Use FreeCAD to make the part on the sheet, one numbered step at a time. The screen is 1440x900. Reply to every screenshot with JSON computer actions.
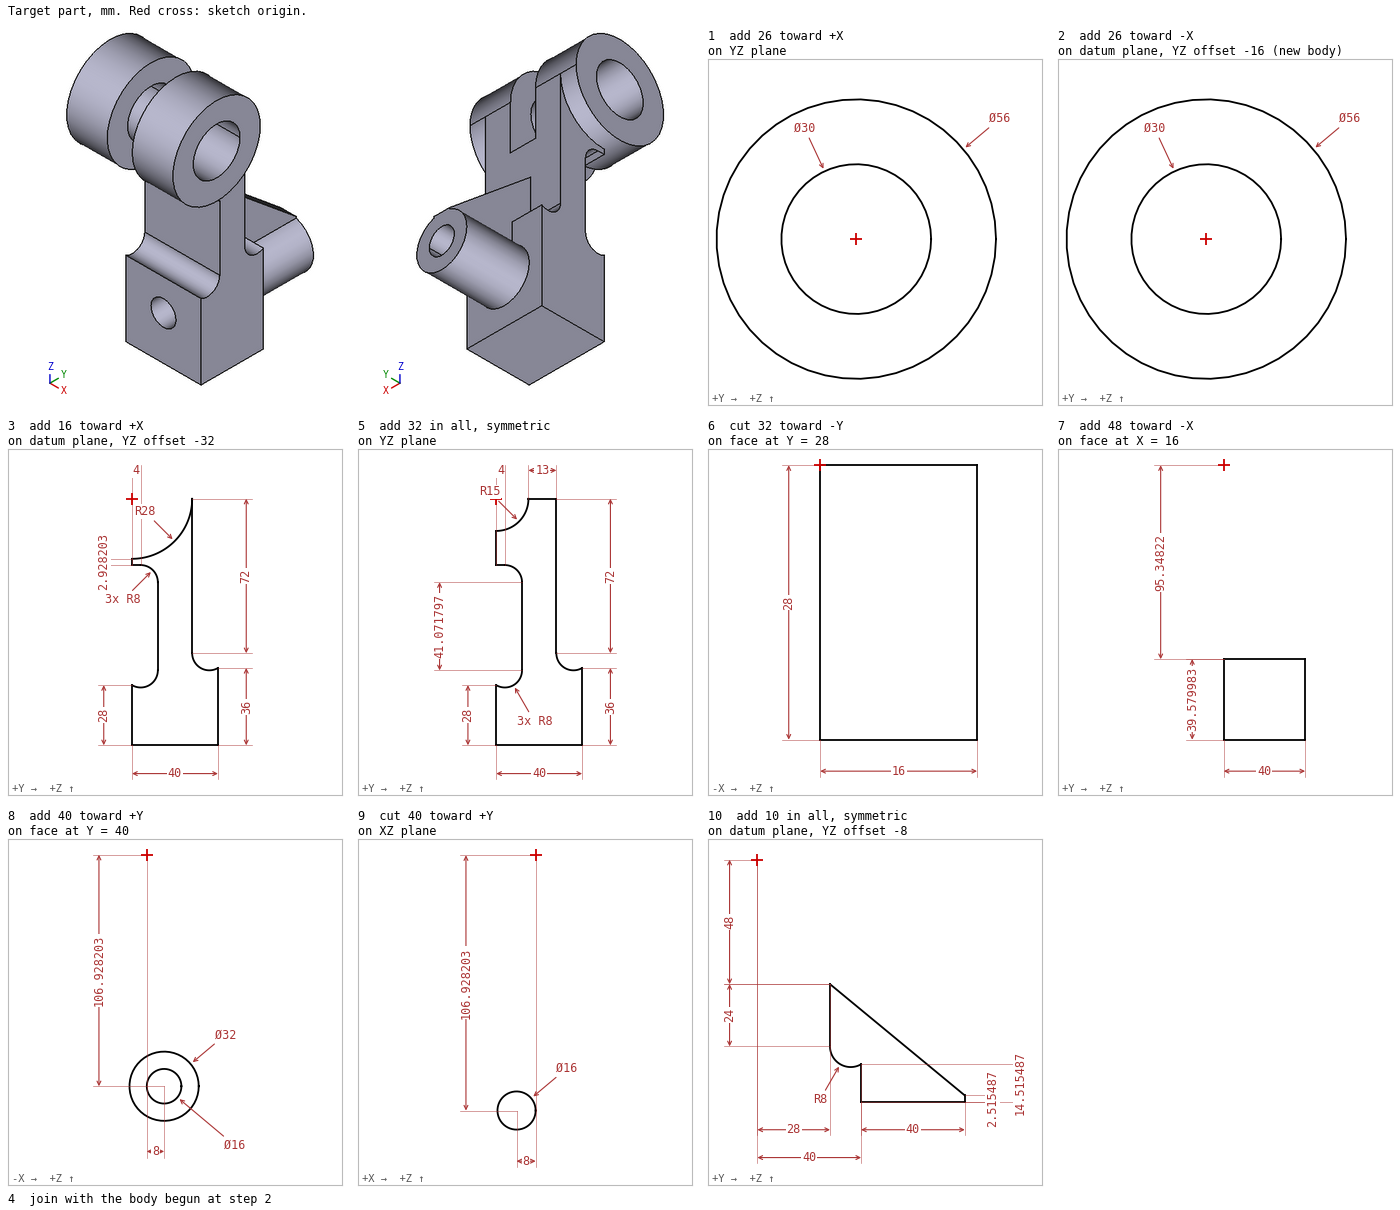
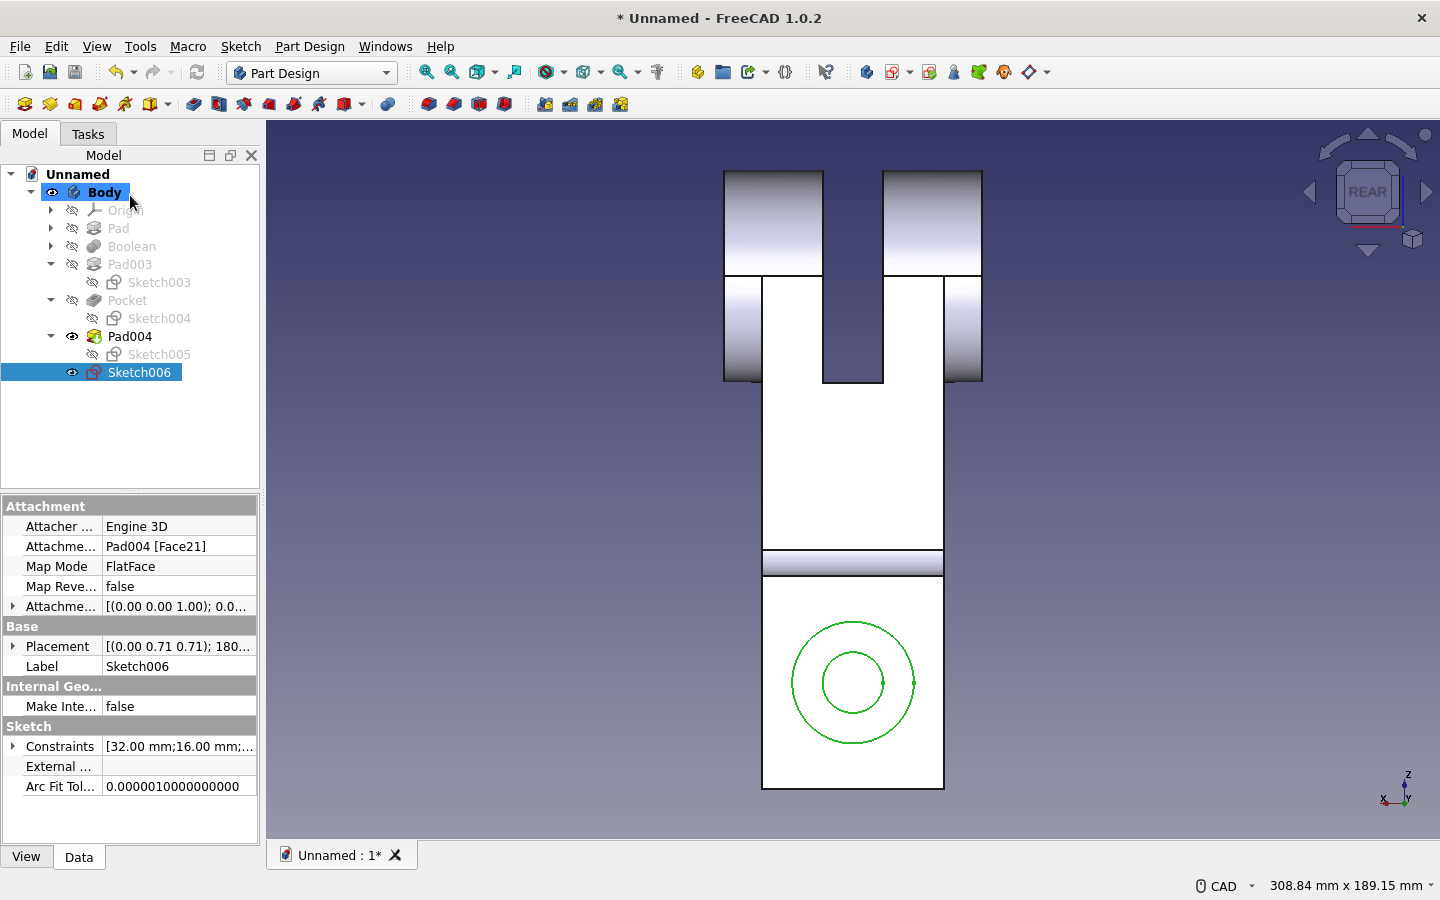
{"action": "left_click", "coordinate": [25, 104]}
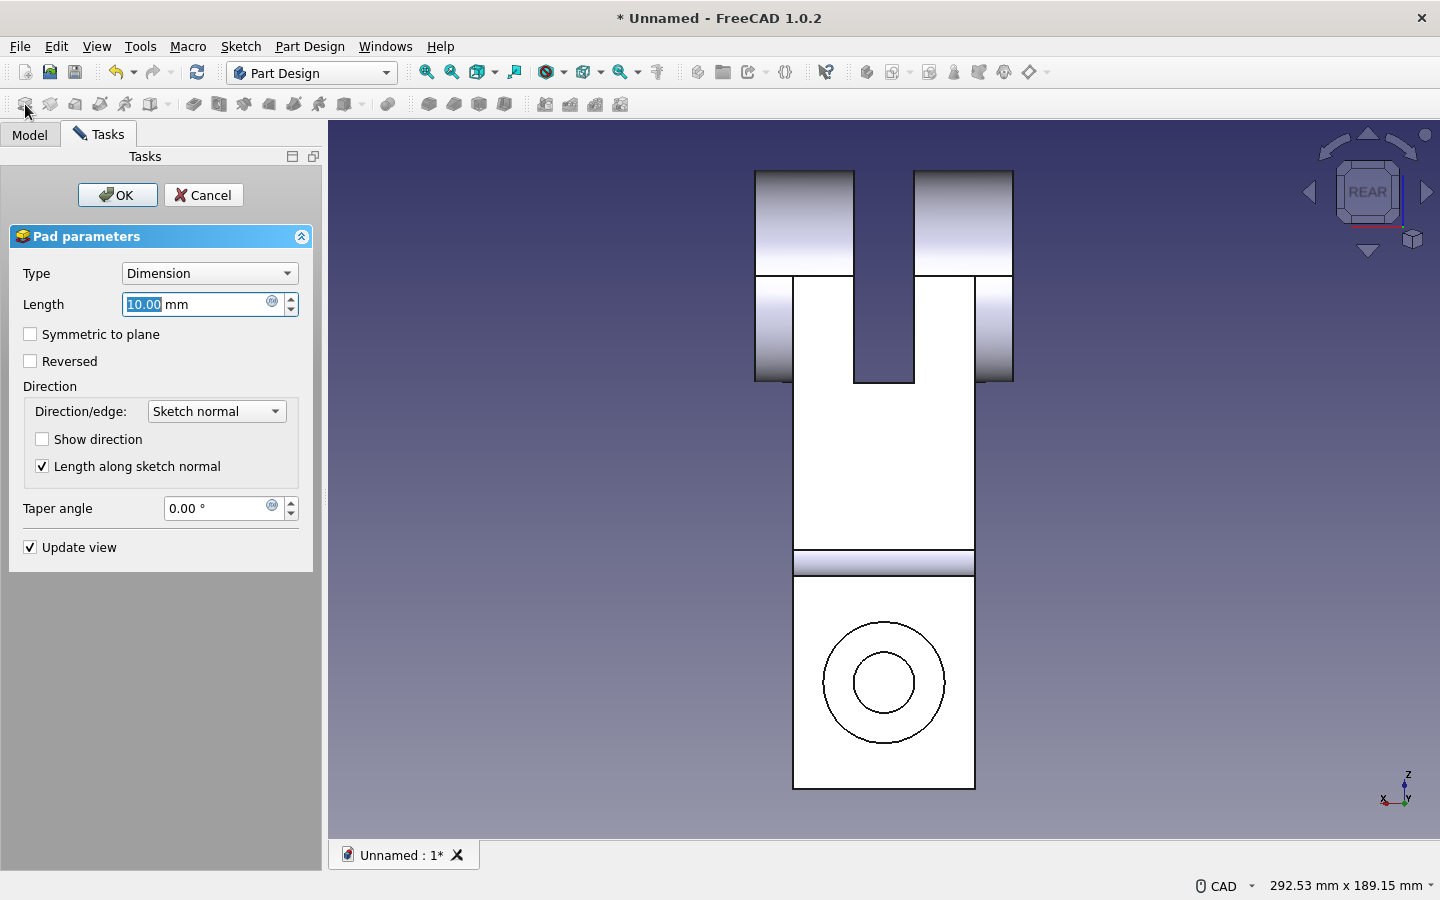
{"action": "type", "text": "40"}
{"action": "key", "text": "Tab"}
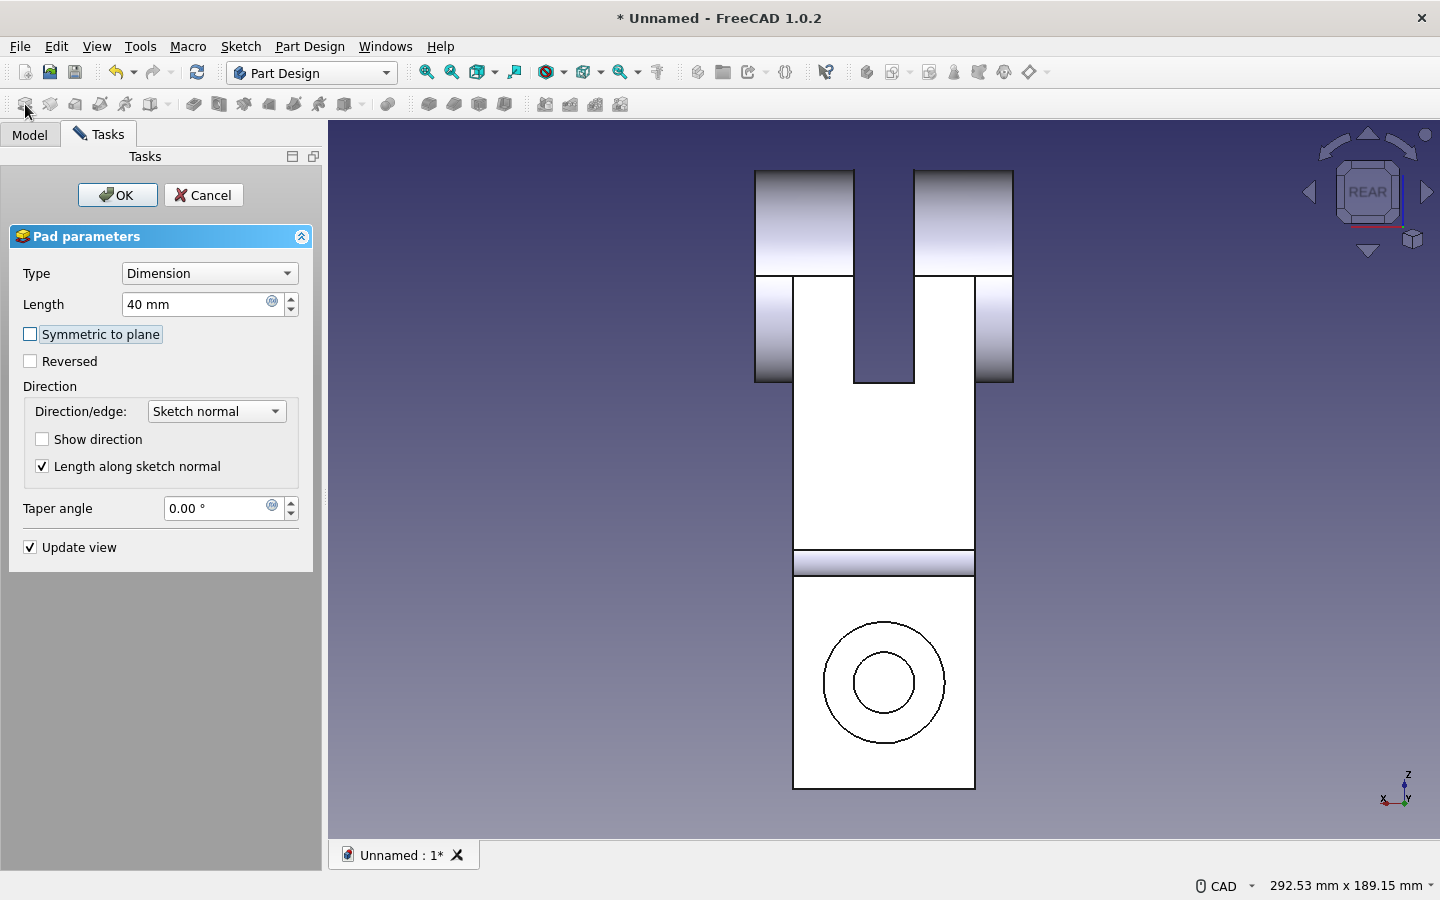
{"action": "left_click", "coordinate": [118, 195]}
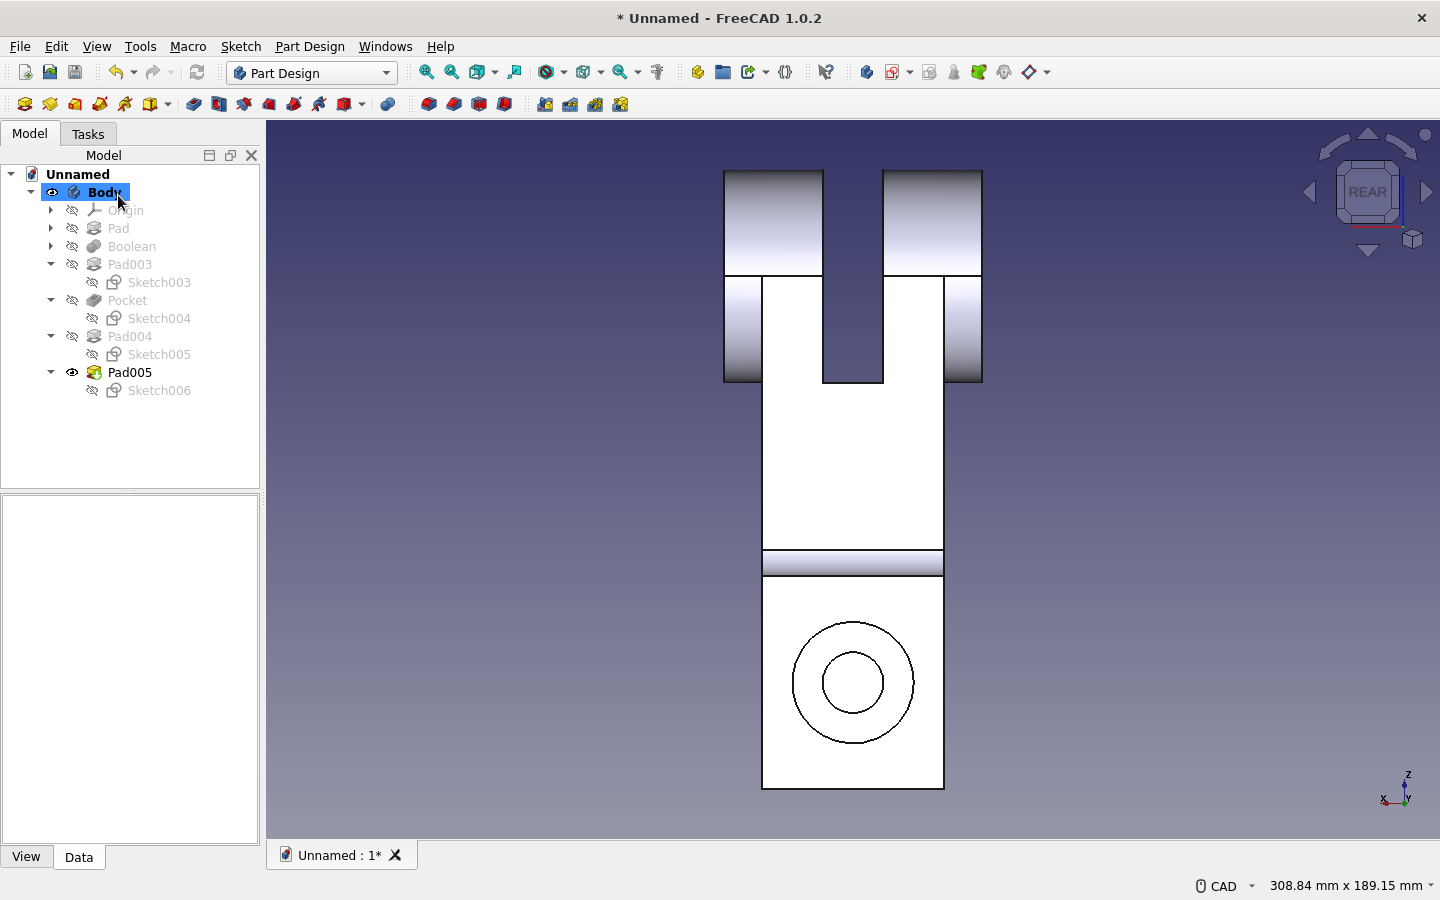
{"action": "left_click", "coordinate": [892, 72]}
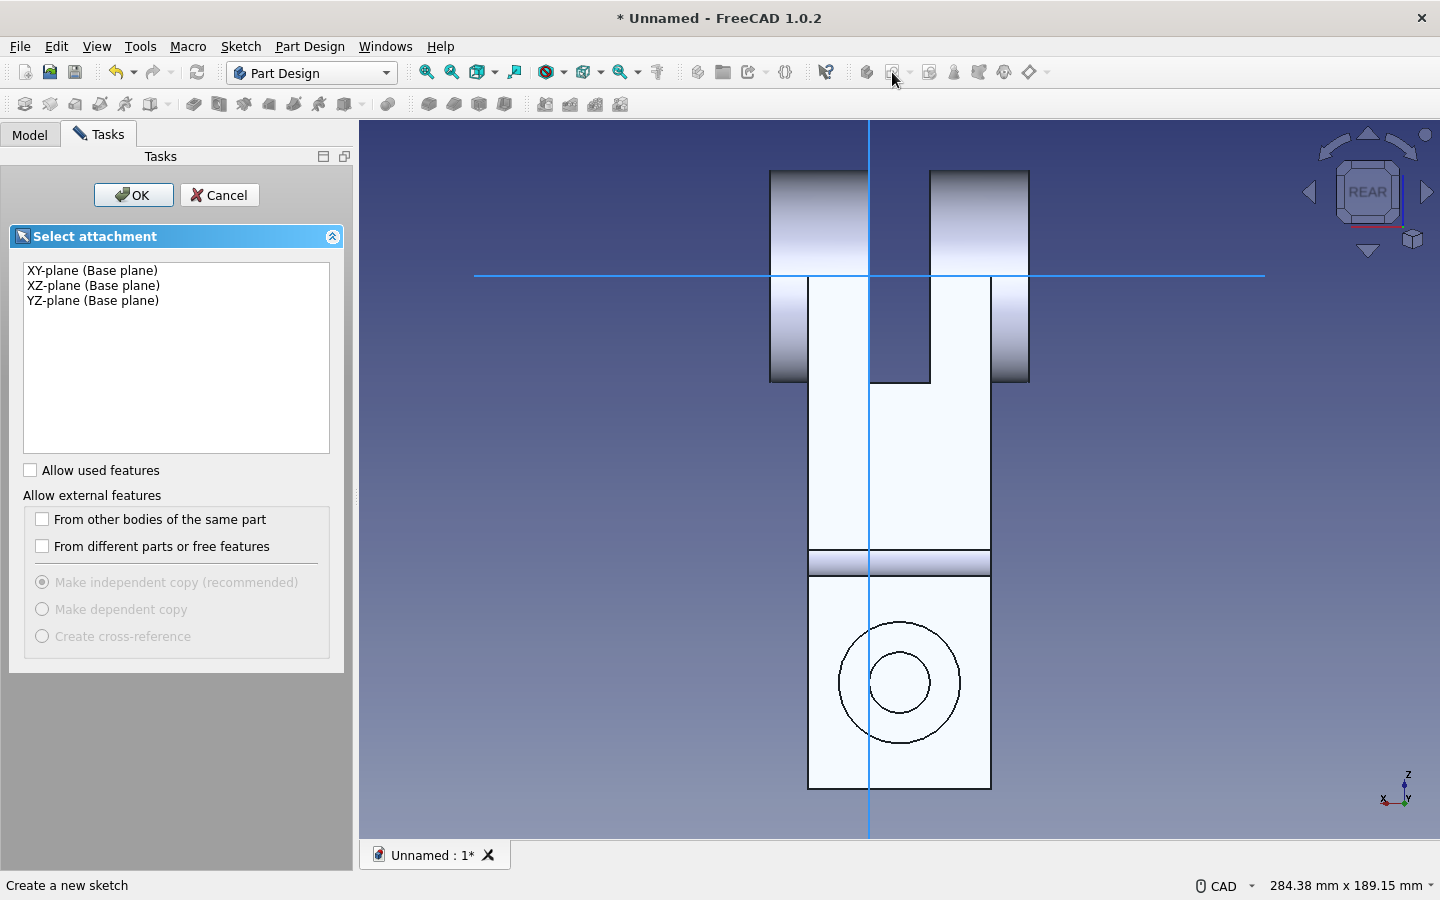
{"action": "left_click", "coordinate": [84, 286]}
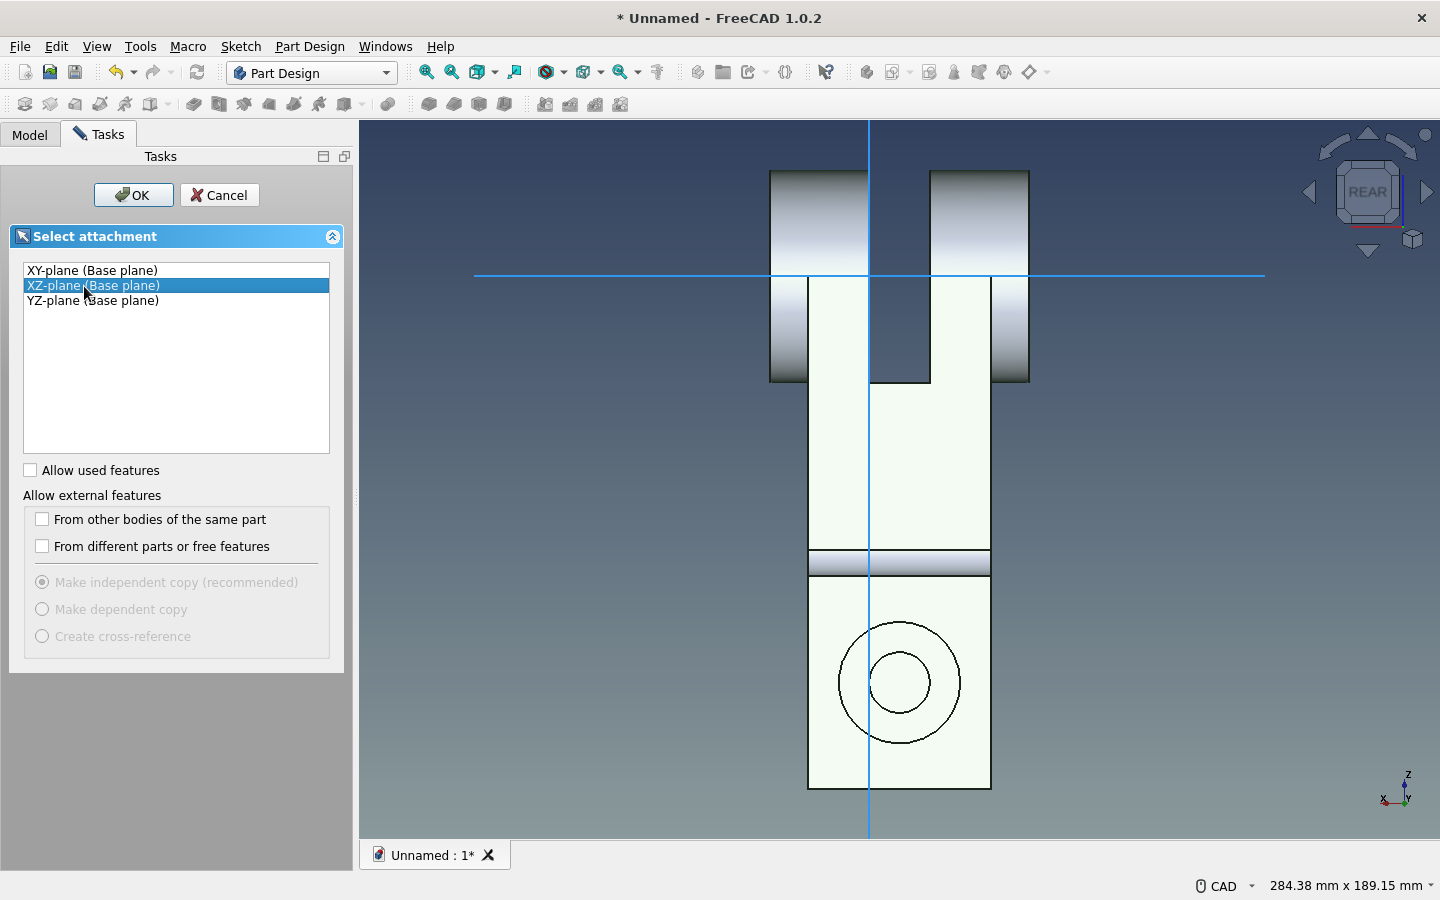
{"action": "left_click", "coordinate": [134, 195]}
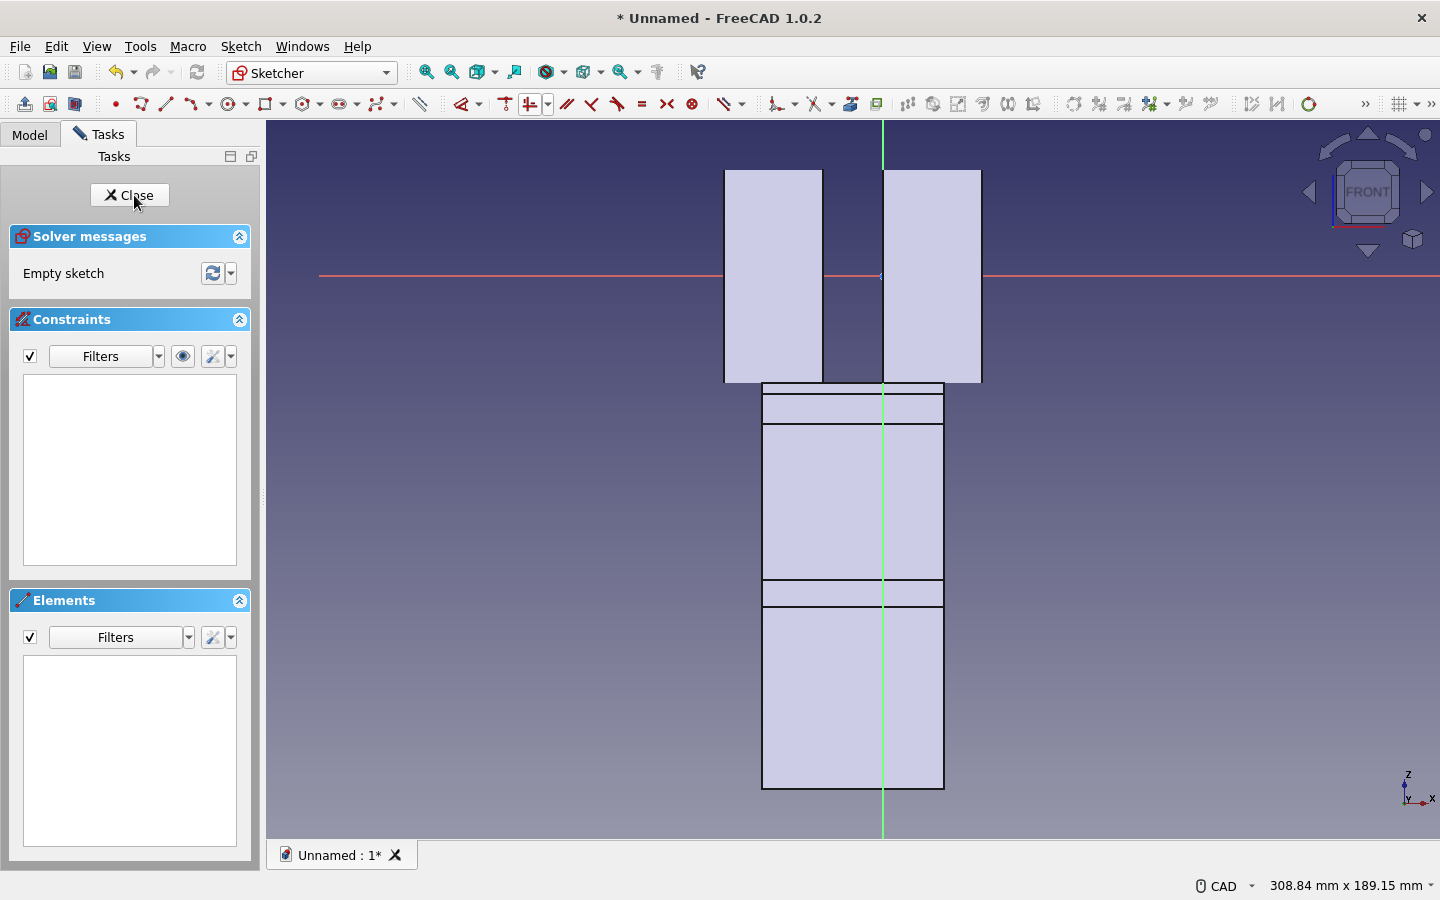
{"action": "left_click", "coordinate": [75, 104]}